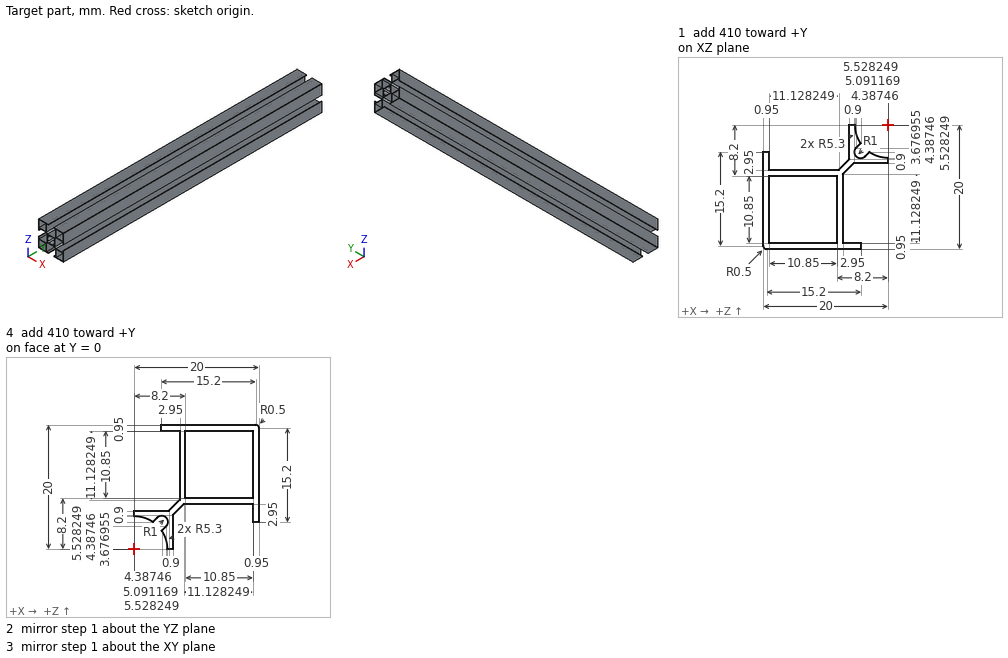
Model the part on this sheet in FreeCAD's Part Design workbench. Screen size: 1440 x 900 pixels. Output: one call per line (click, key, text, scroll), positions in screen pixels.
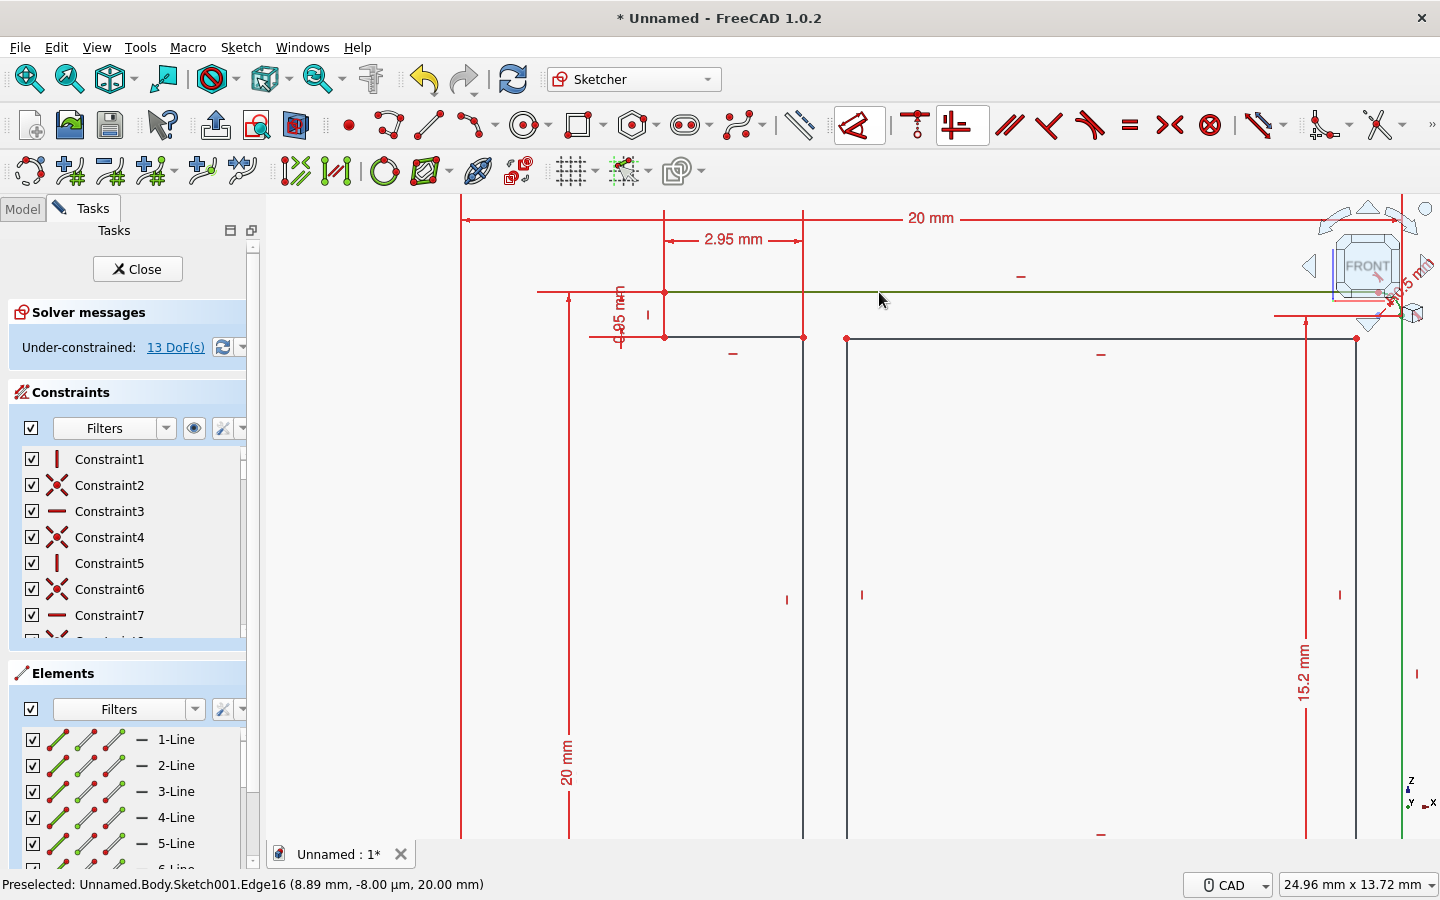
key(l)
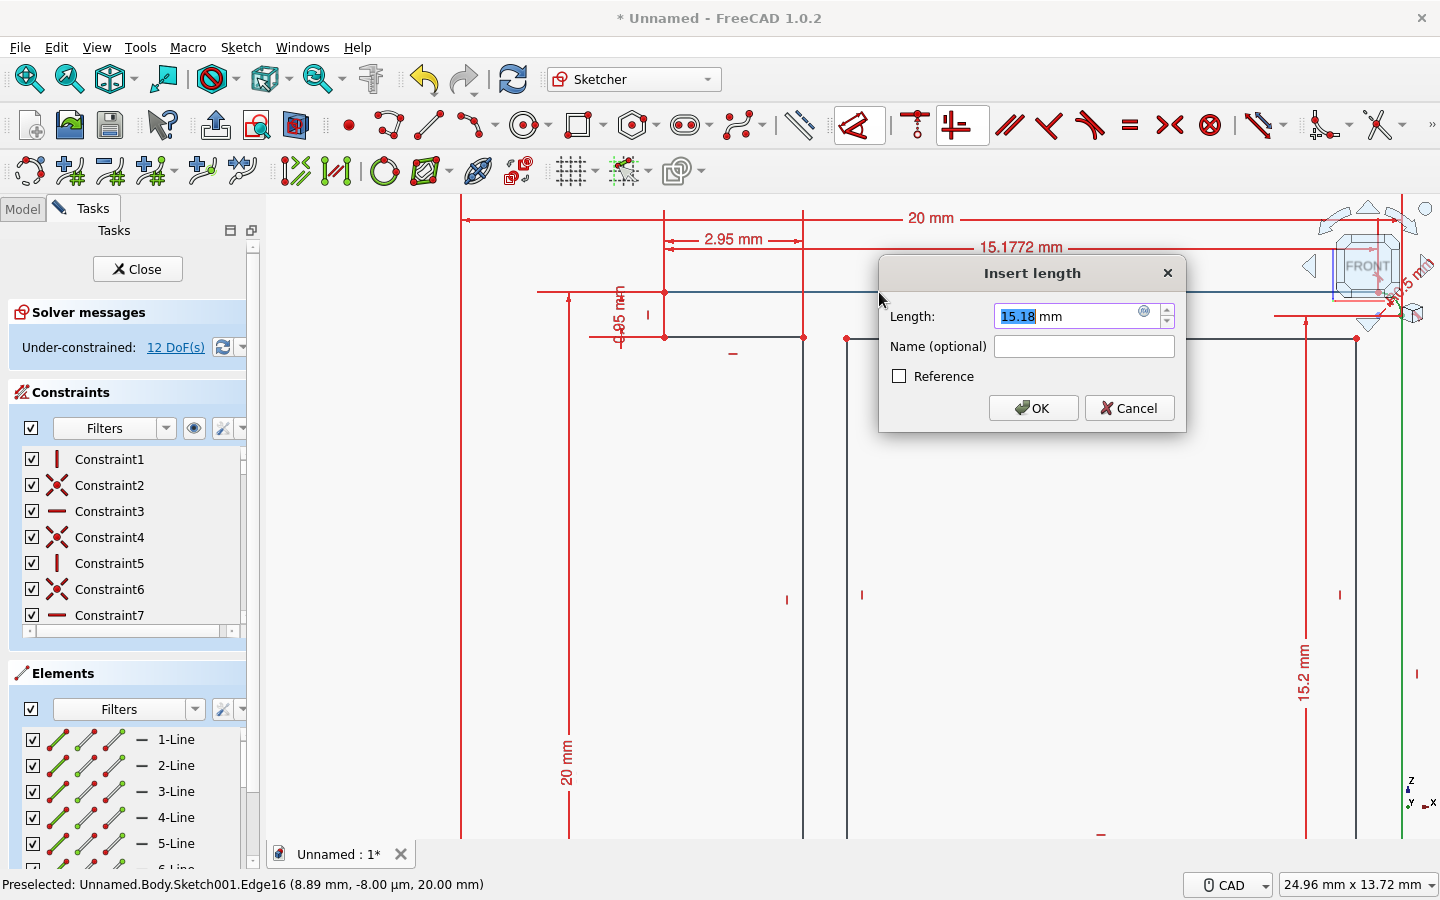
text(15.2)
key(Return)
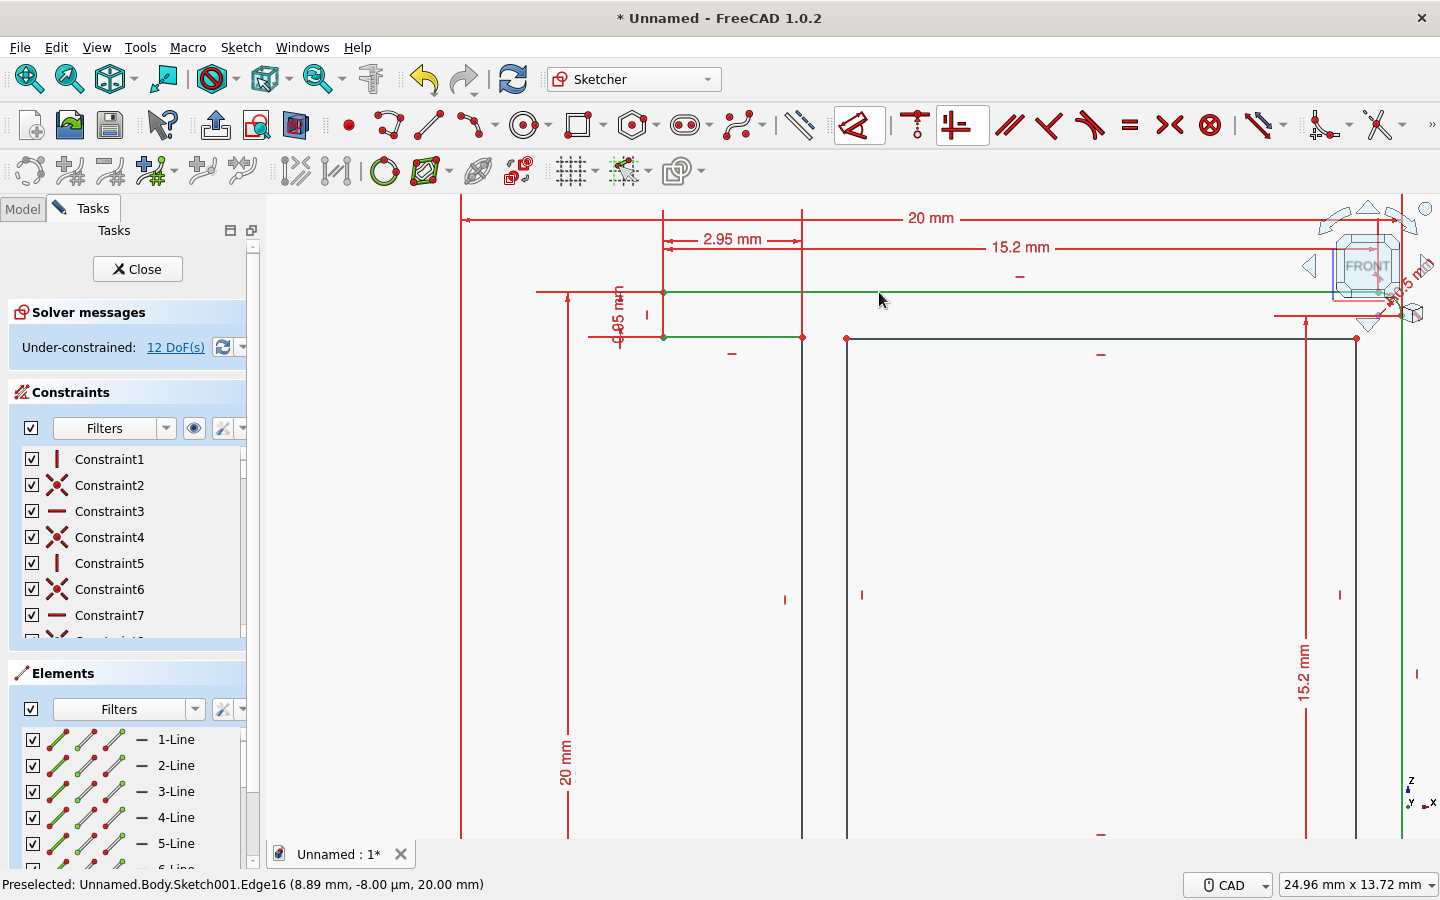
click(847, 339)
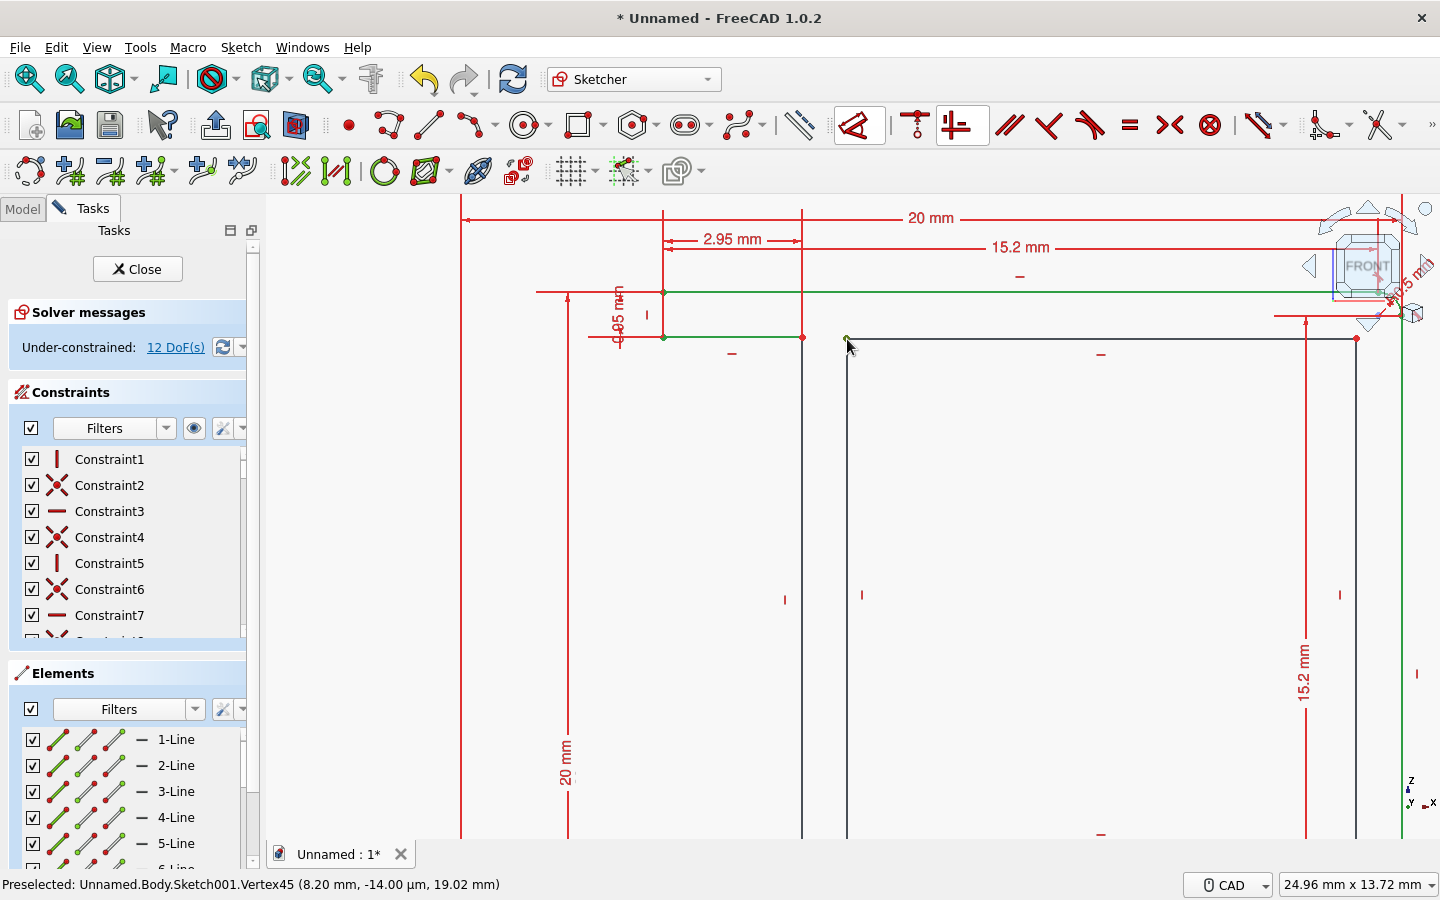
click(880, 126)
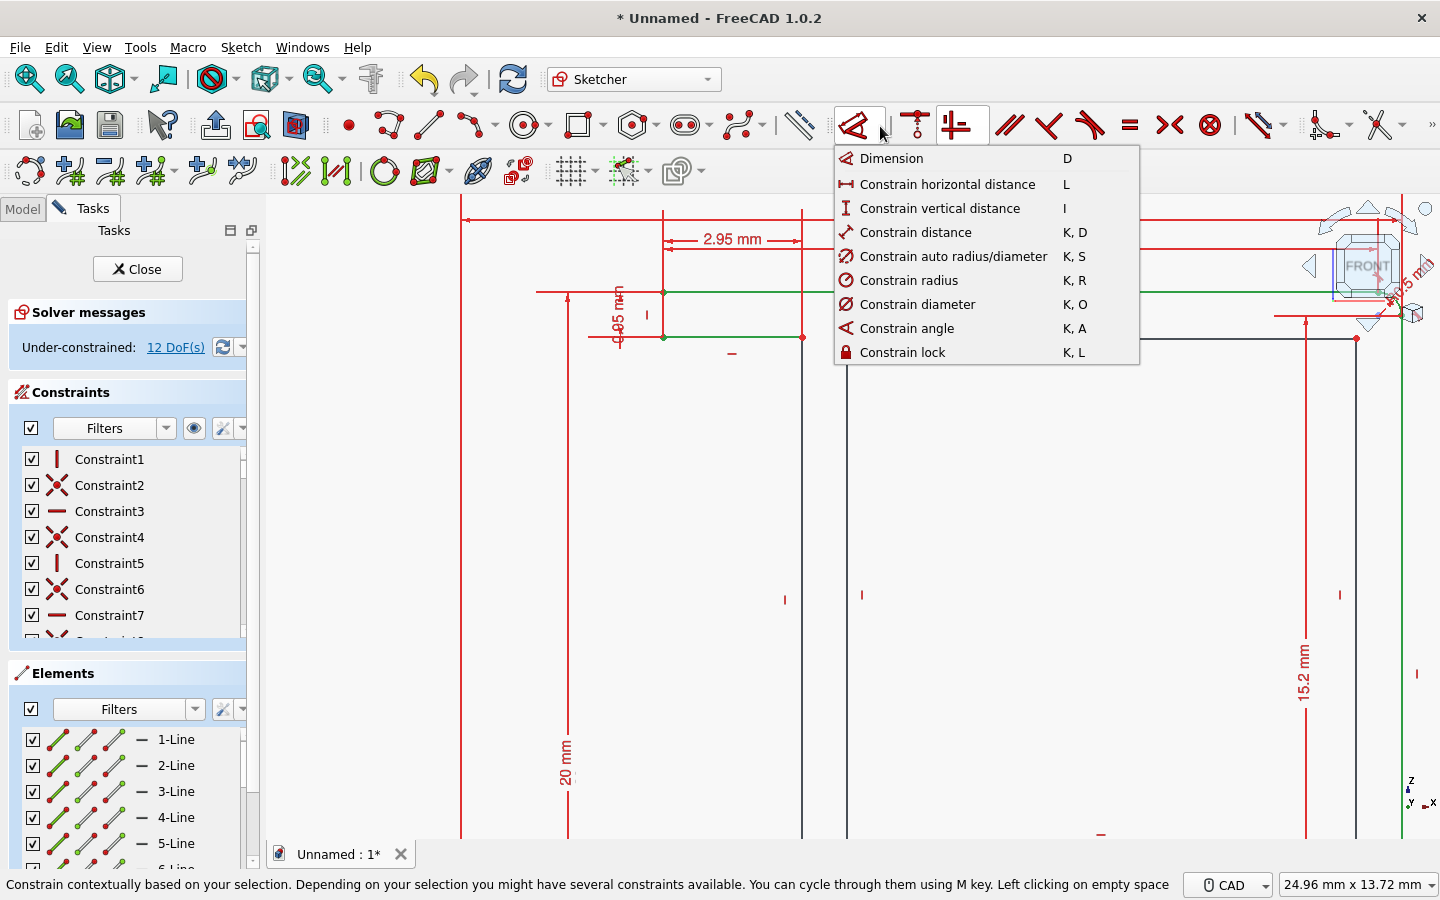
click(987, 184)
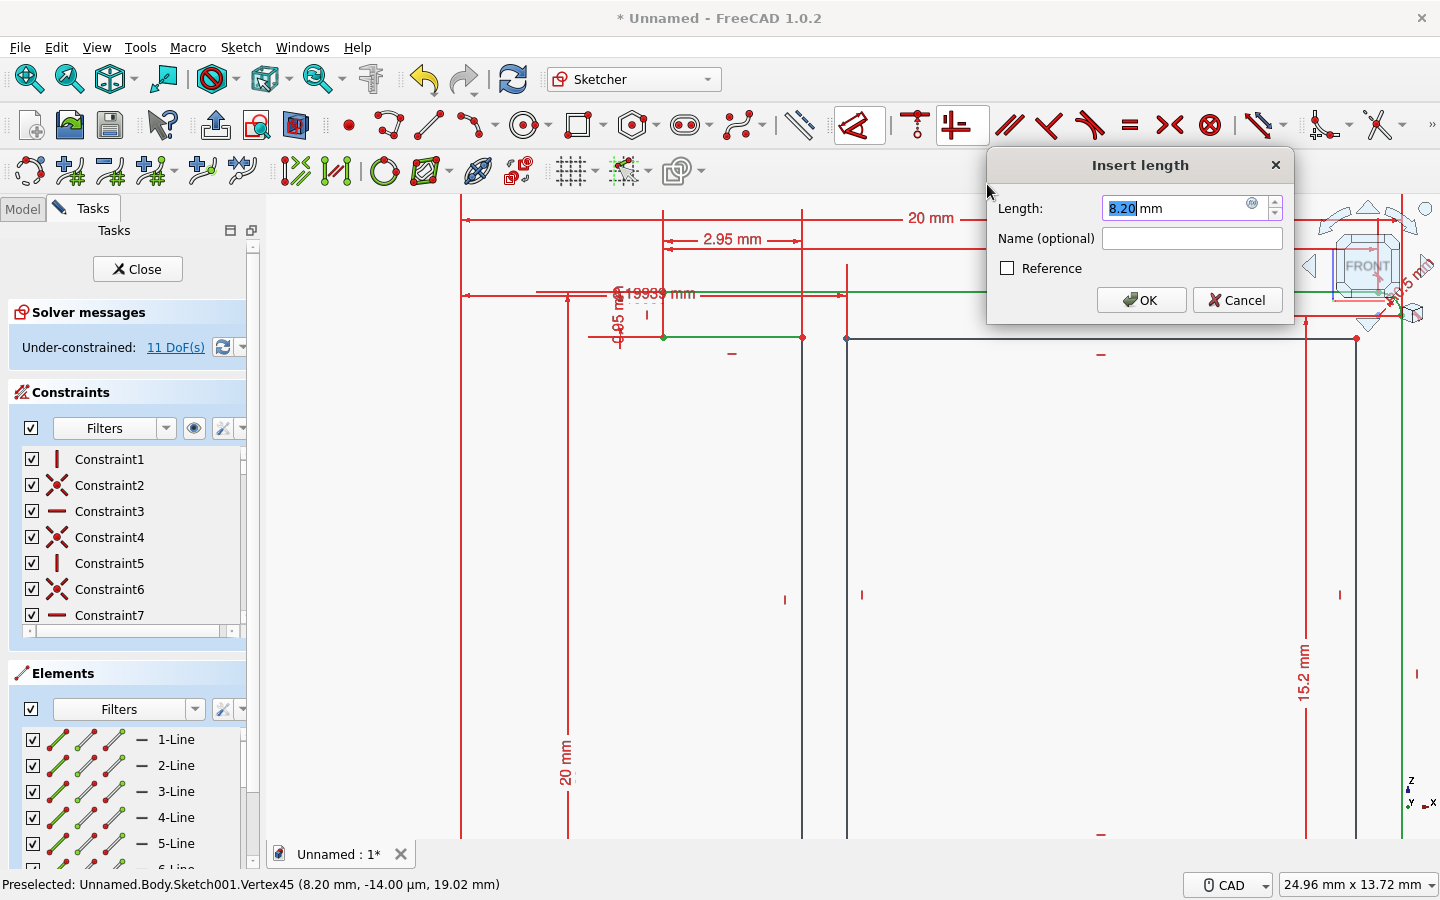
text(8.2)
key(Return)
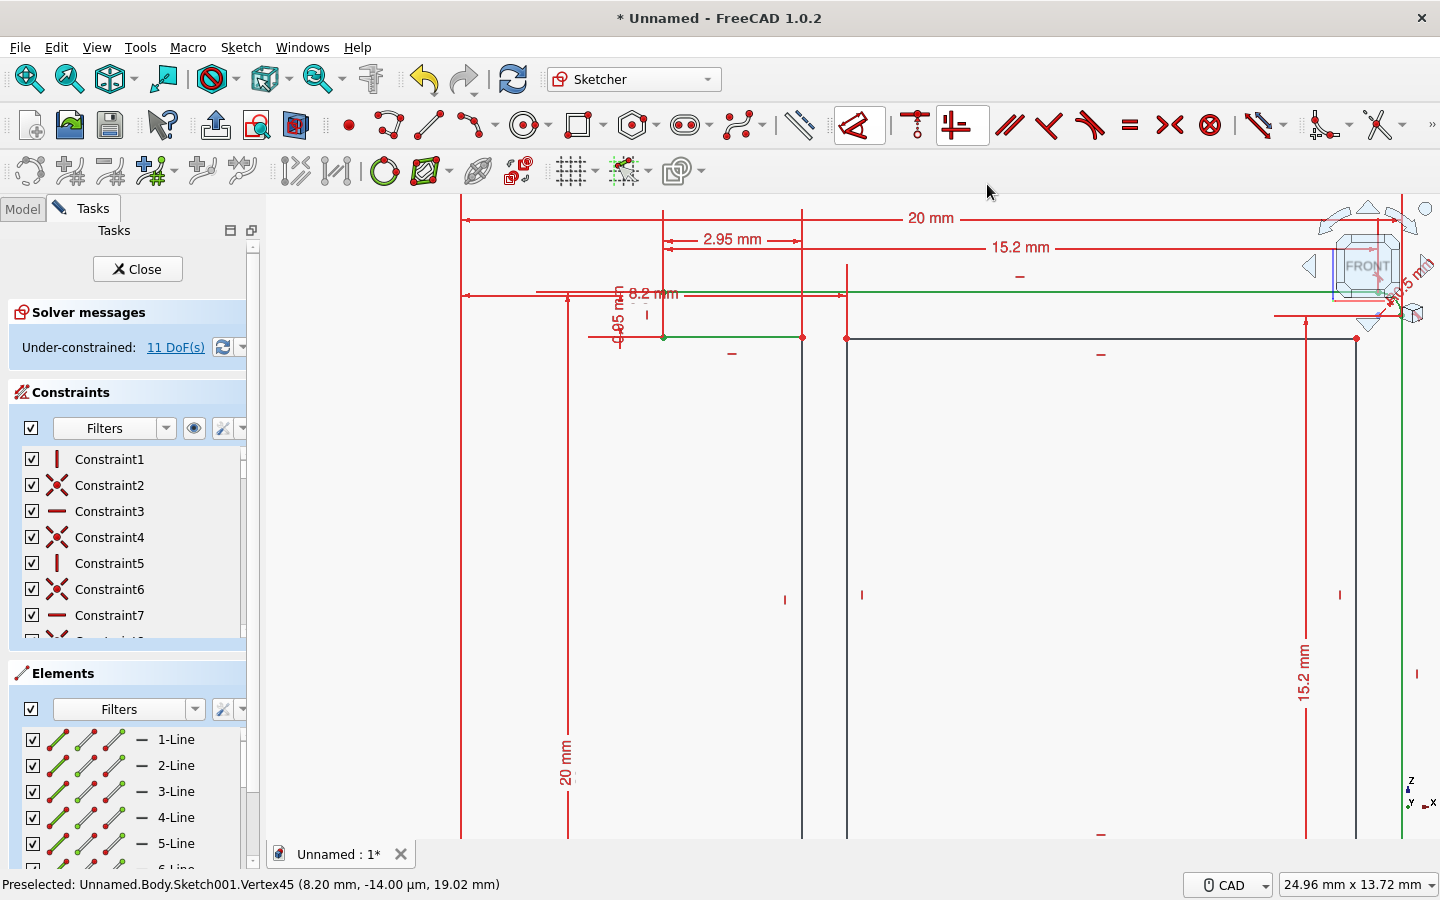
scroll(665, 316, down, 4)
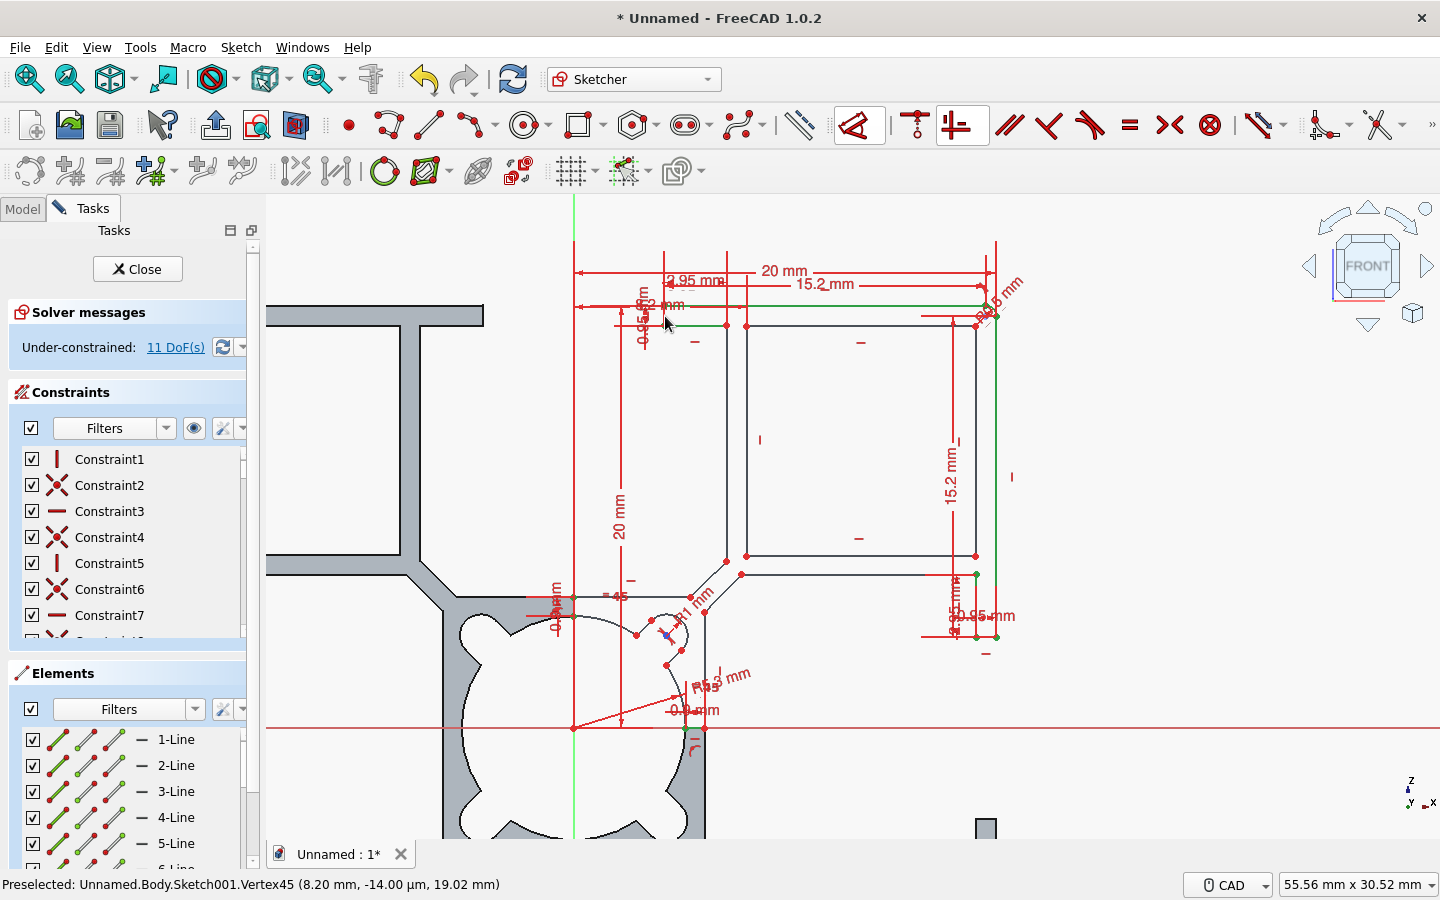
click(747, 556)